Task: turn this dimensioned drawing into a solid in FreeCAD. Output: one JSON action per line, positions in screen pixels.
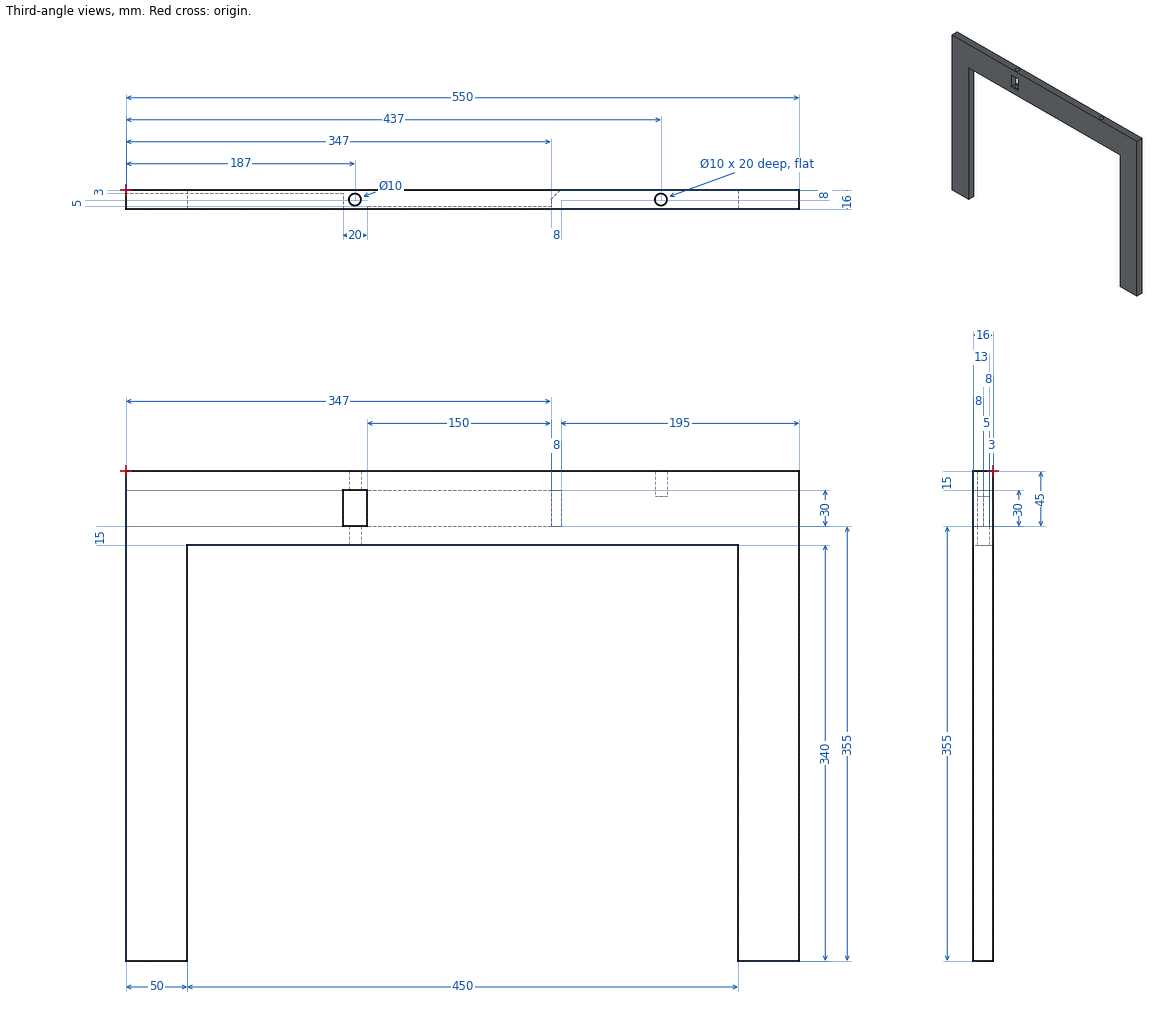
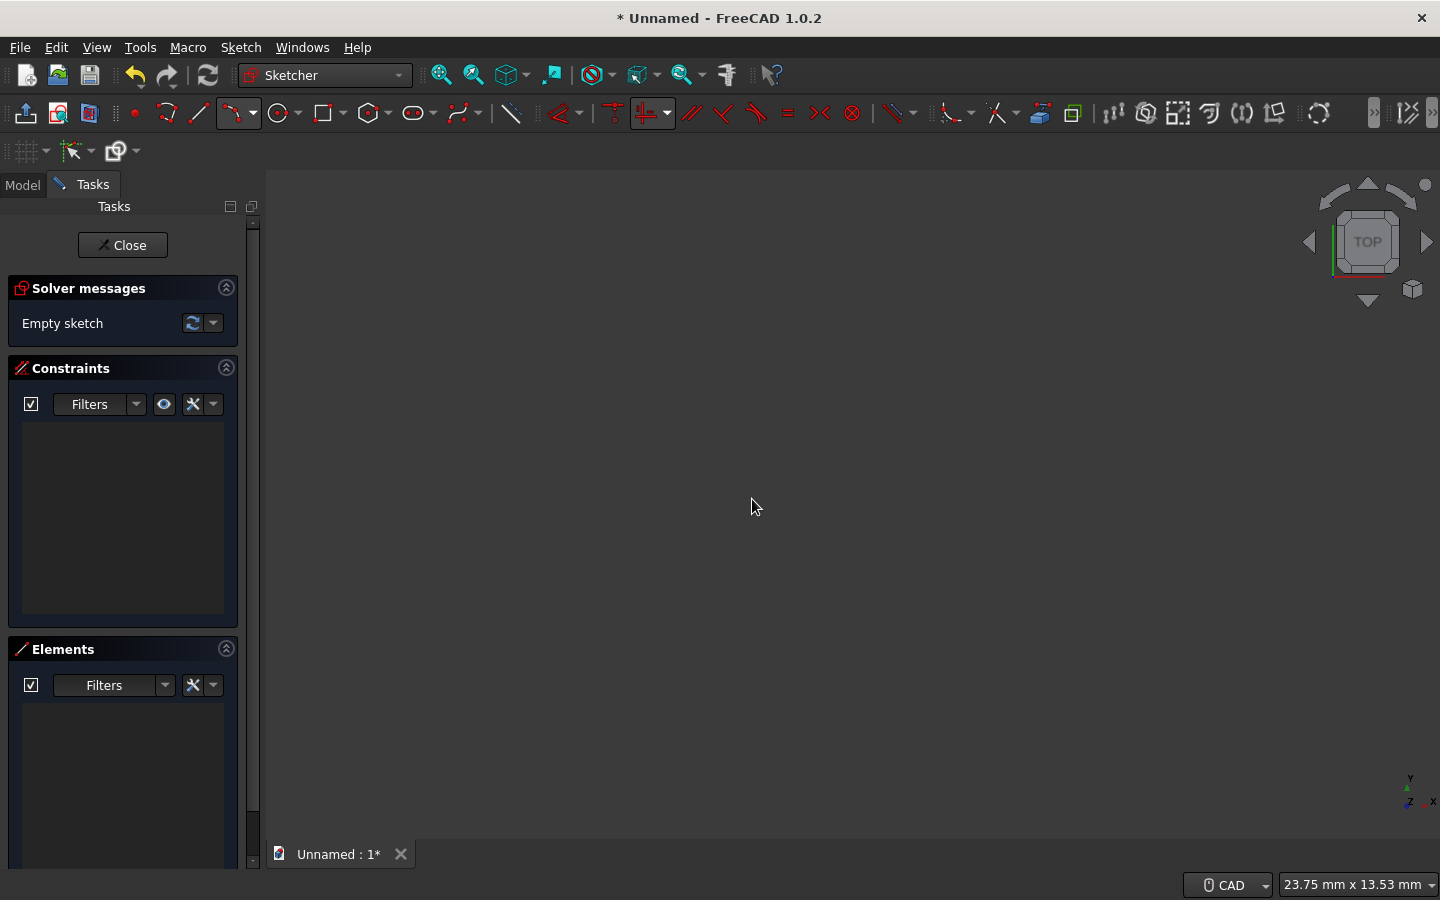
{"action": "left_click", "coordinate": [168, 114]}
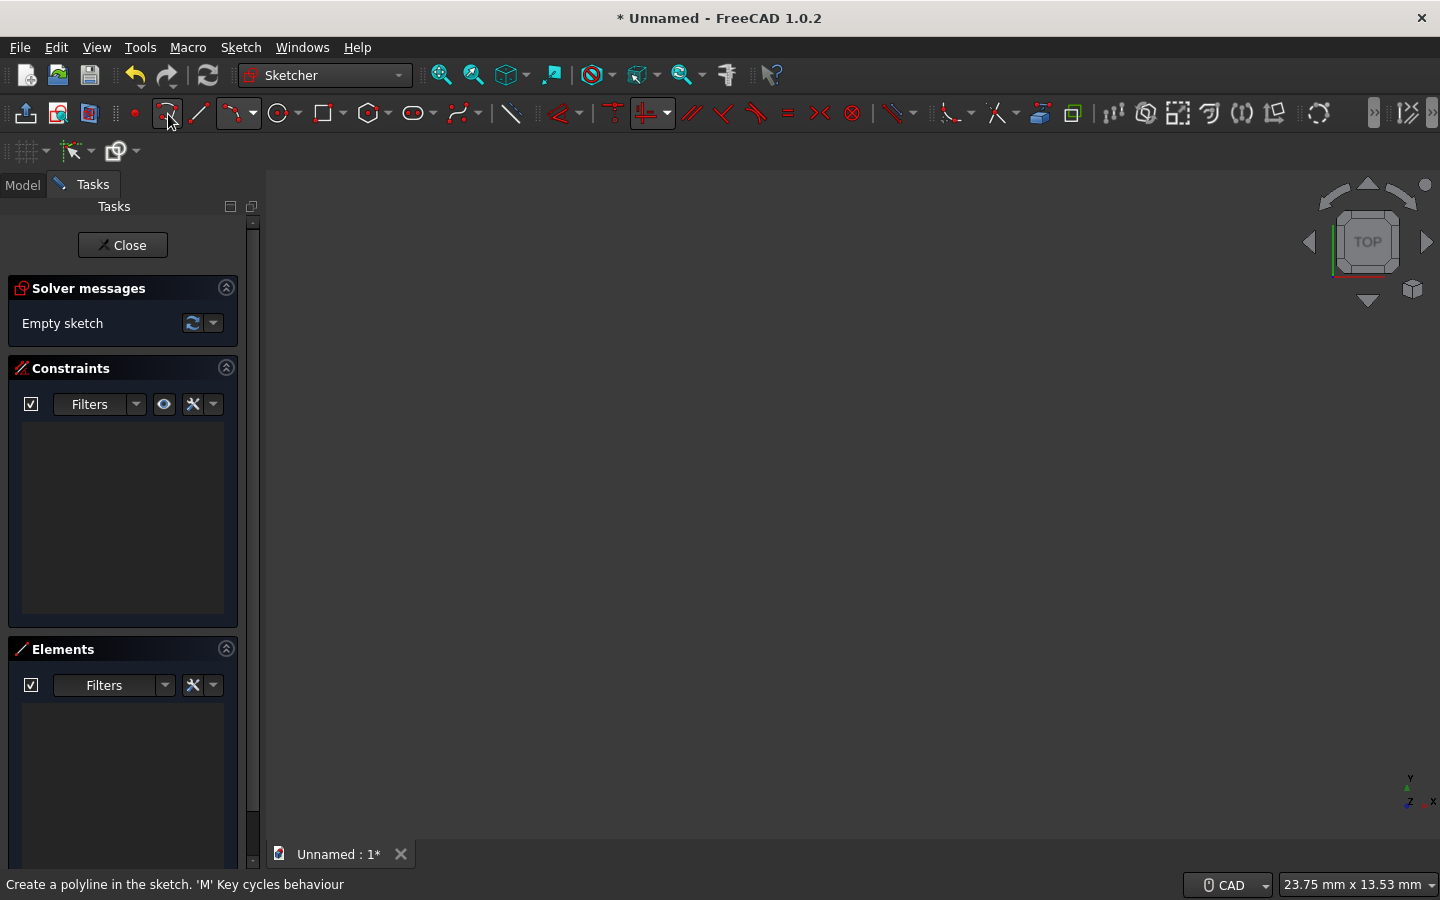
{"action": "left_click", "coordinate": [585, 701]}
{"action": "left_click", "coordinate": [981, 305]}
{"action": "left_click", "coordinate": [981, 701]}
{"action": "left_click", "coordinate": [585, 702]}
{"action": "key", "text": "Escape"}
{"action": "key", "text": "Escape"}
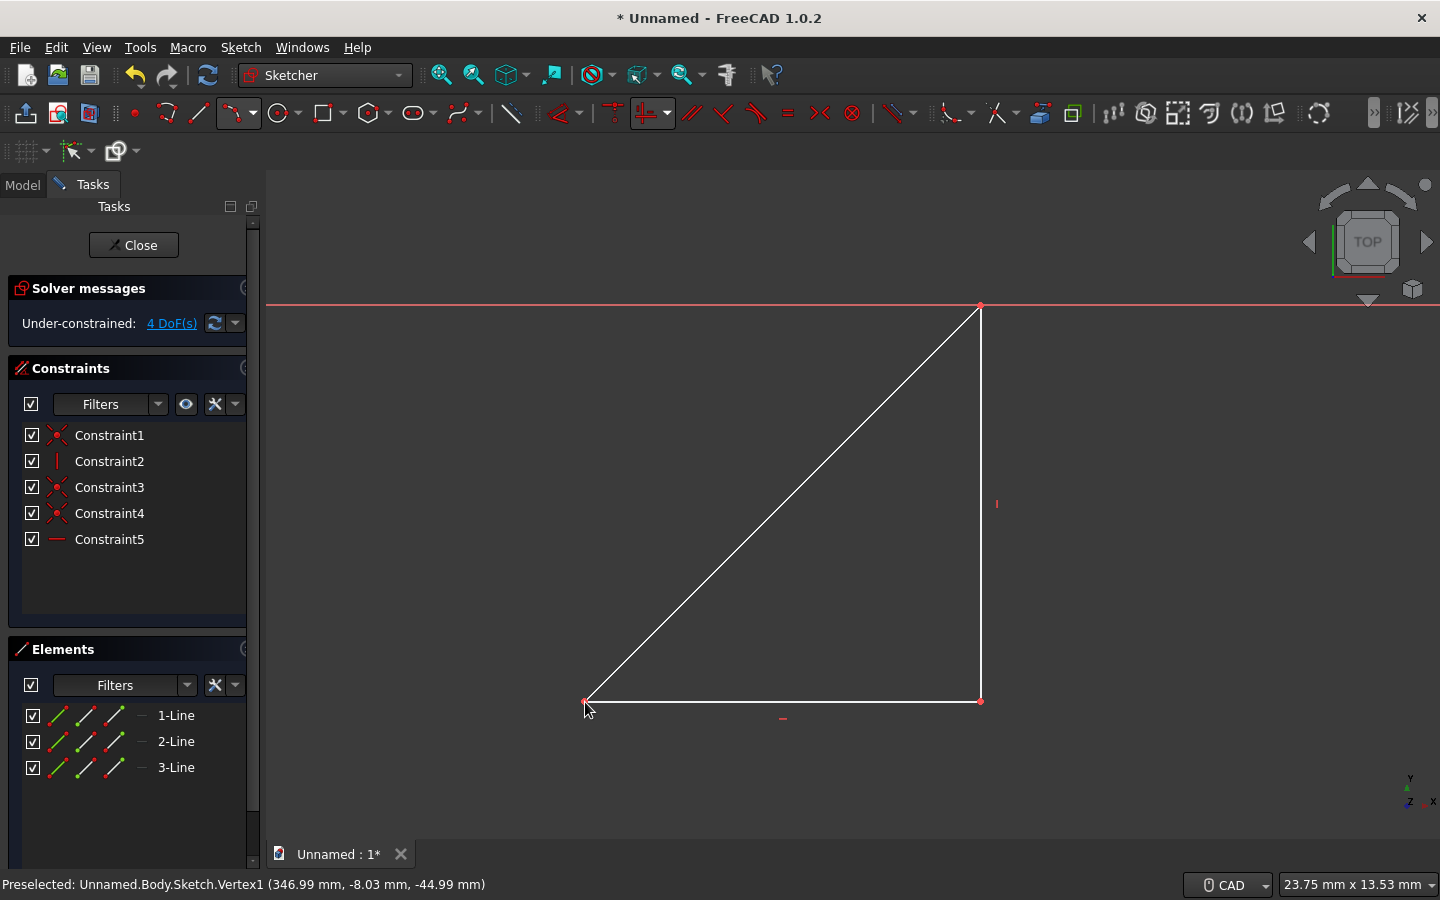
{"action": "left_click", "coordinate": [981, 306]}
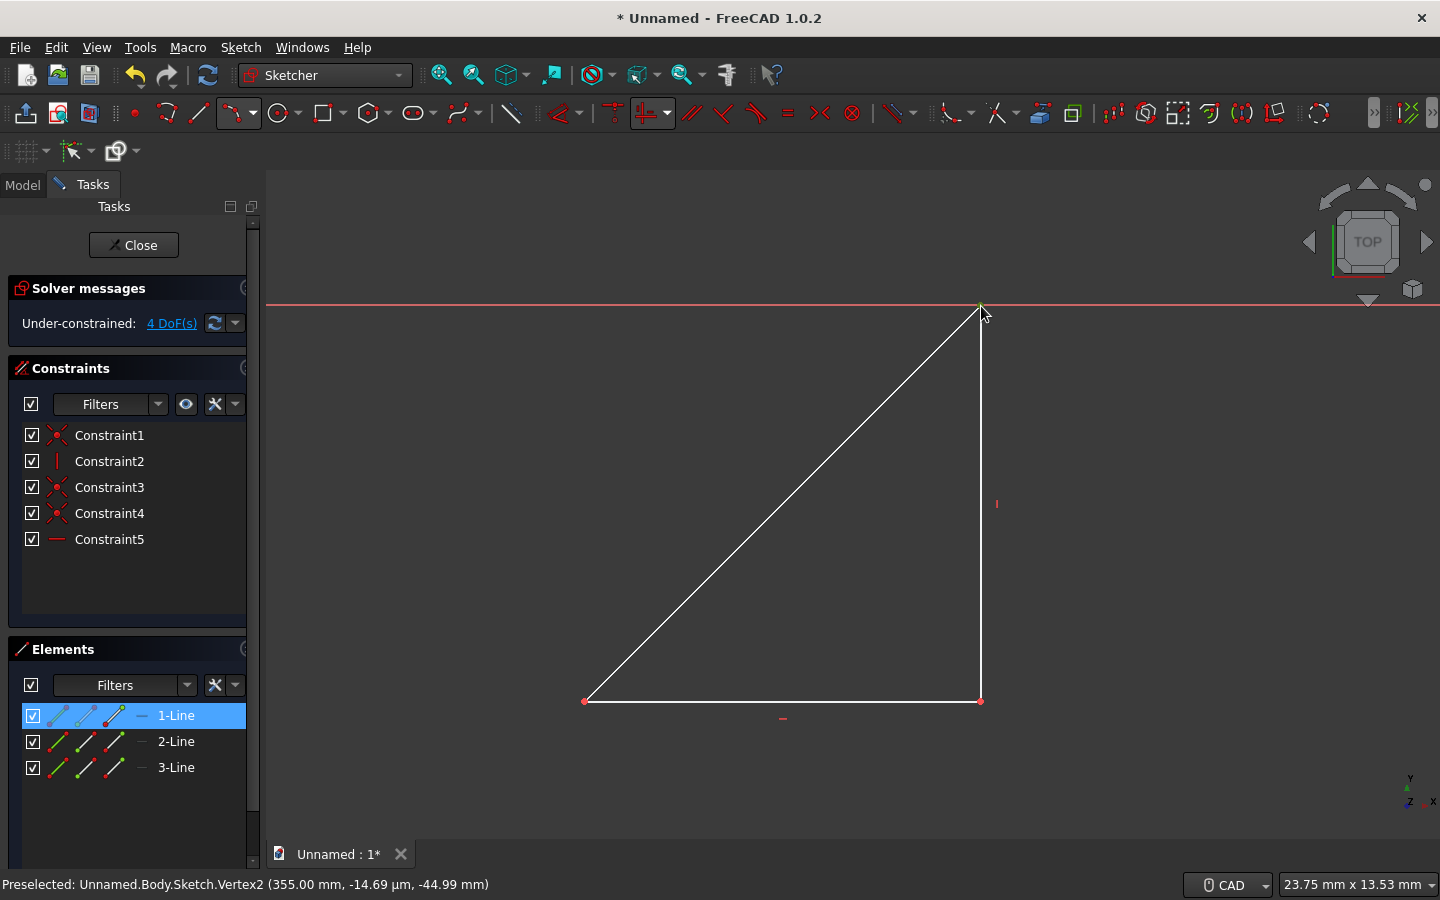
{"action": "left_click", "coordinate": [364, 305]}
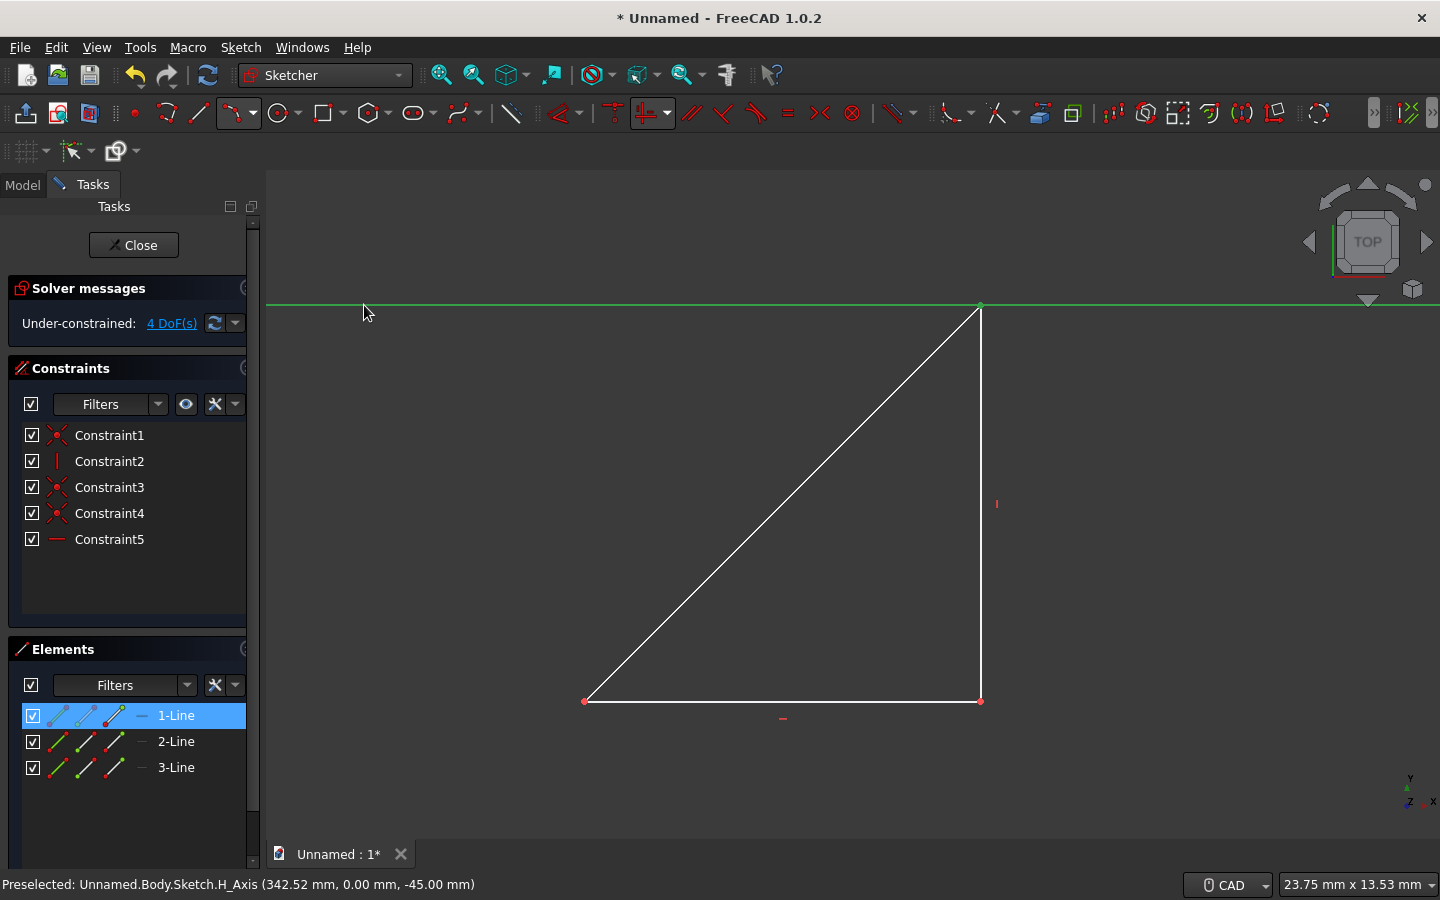
{"action": "left_click", "coordinate": [614, 114]}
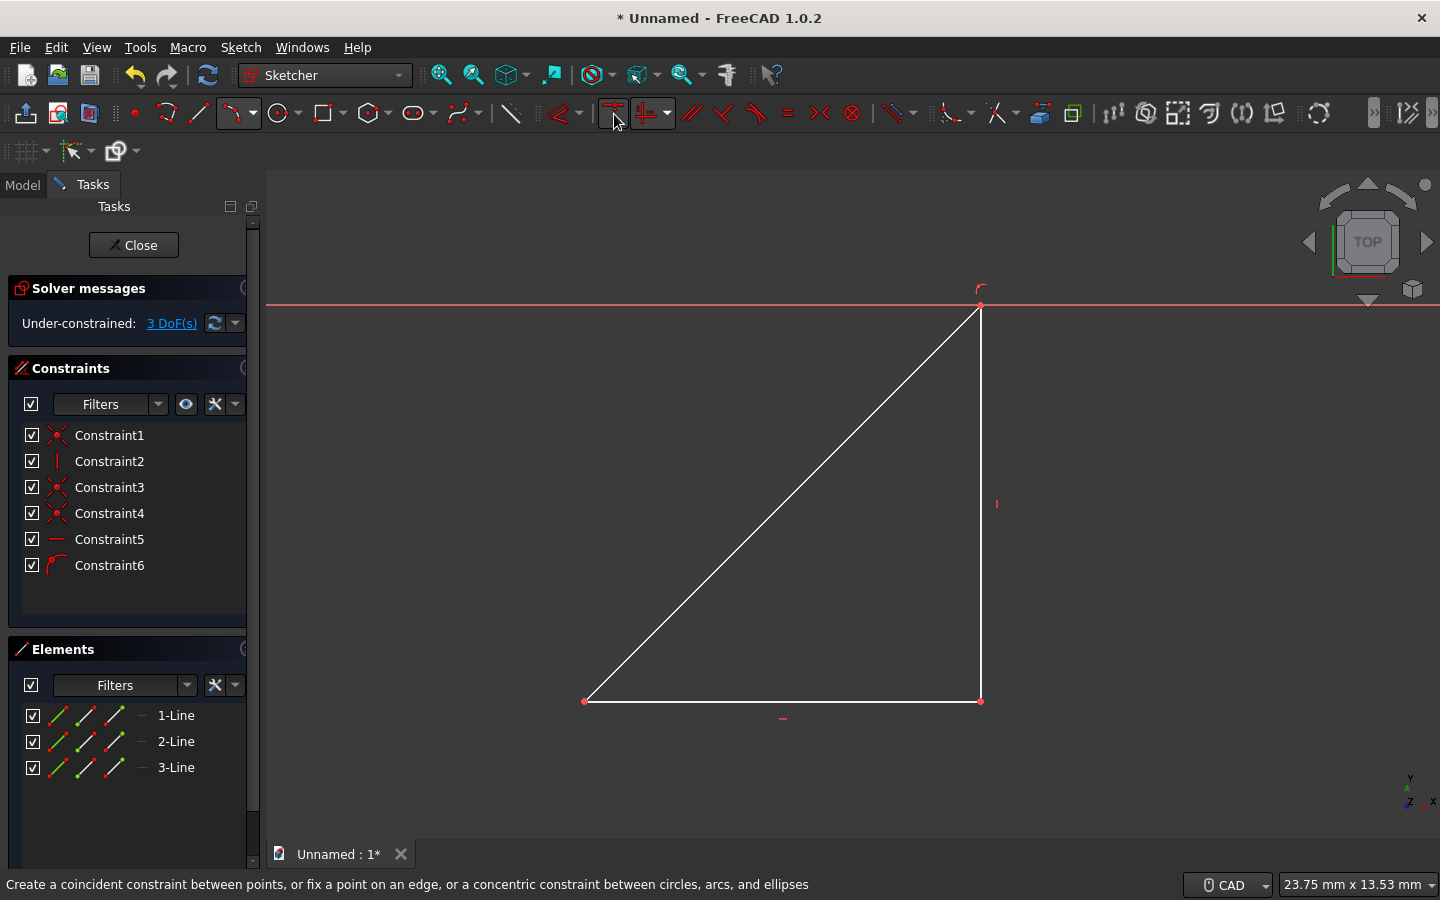
{"action": "left_click", "coordinate": [981, 424]}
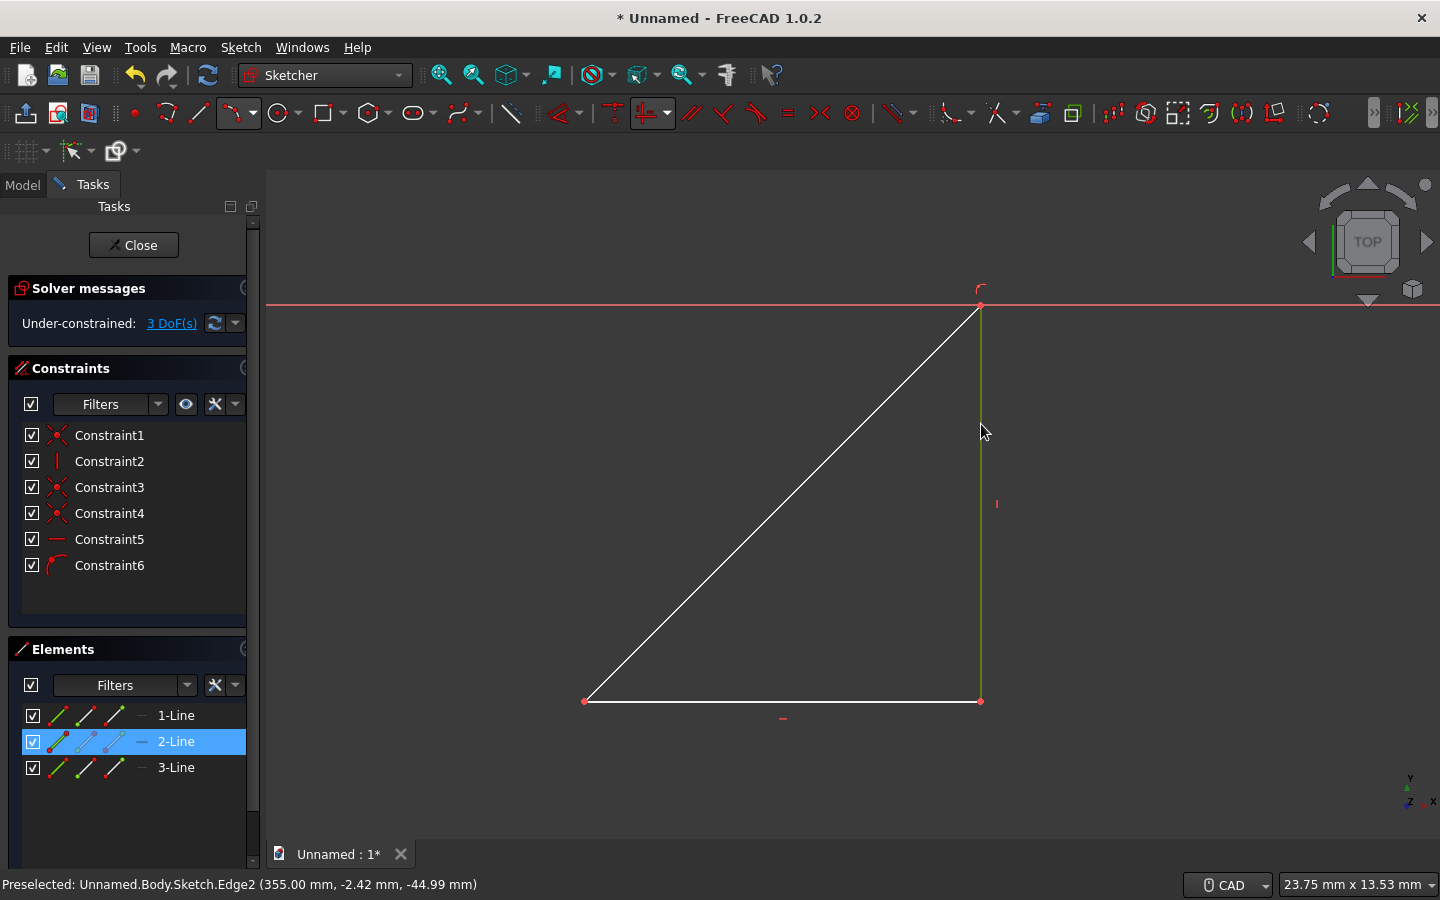
{"action": "left_click", "coordinate": [582, 114]}